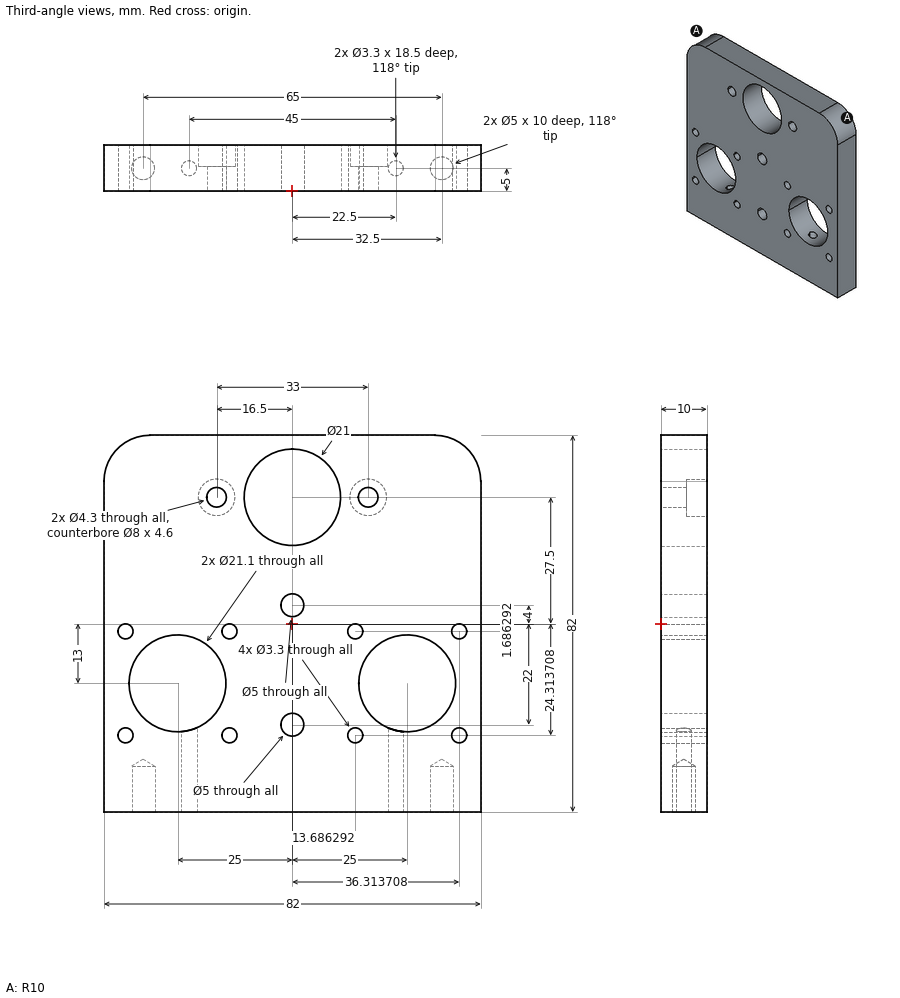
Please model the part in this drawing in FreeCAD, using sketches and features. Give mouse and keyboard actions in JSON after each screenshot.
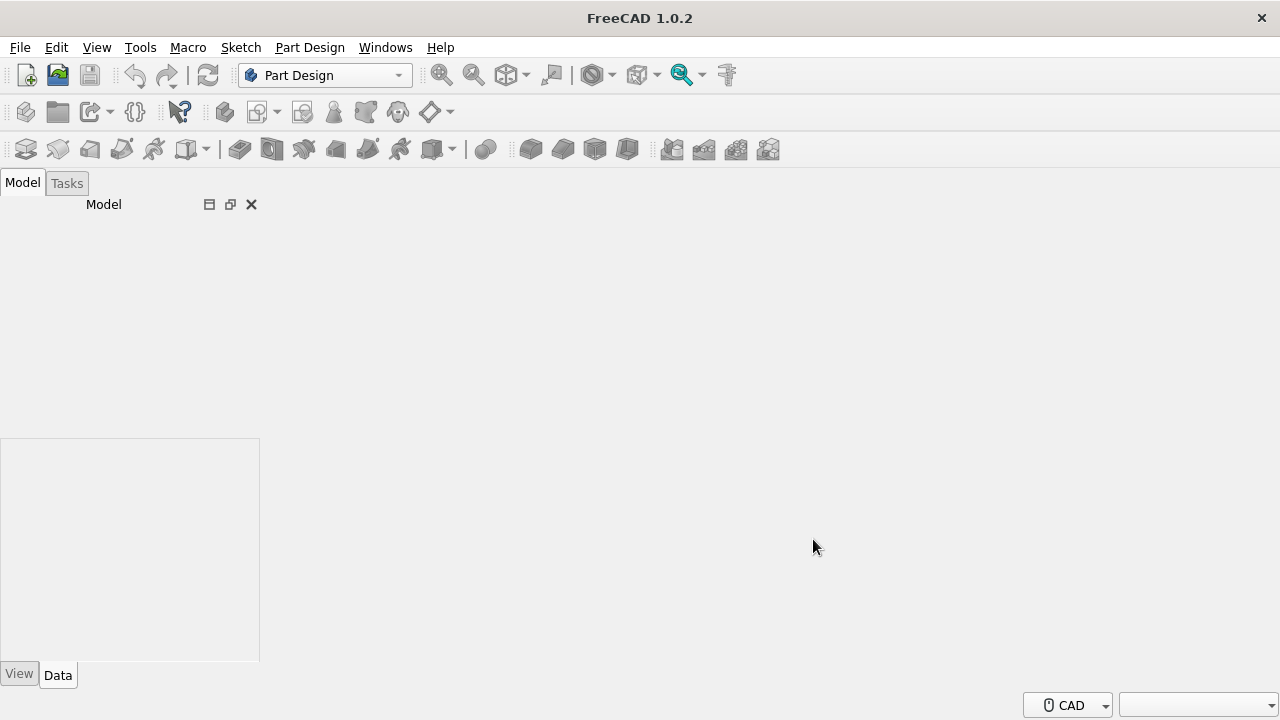
{"action": "left_click", "coordinate": [26, 76]}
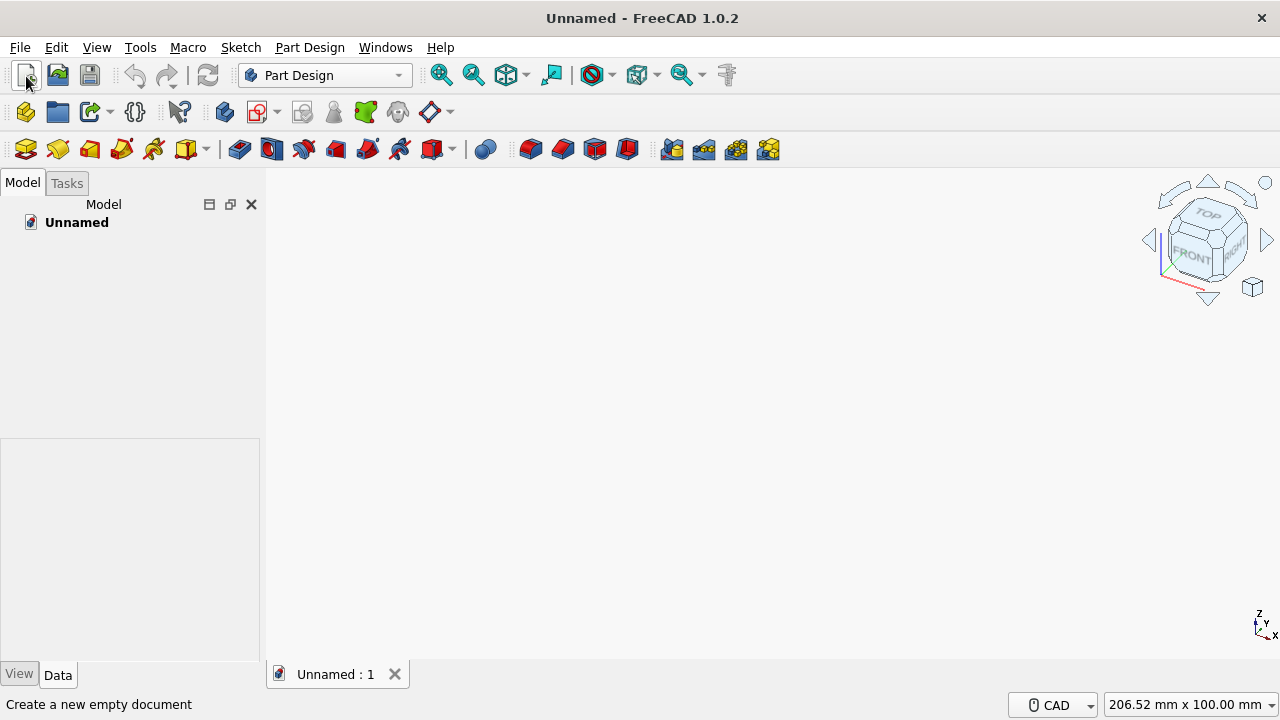
{"action": "left_click", "coordinate": [258, 112]}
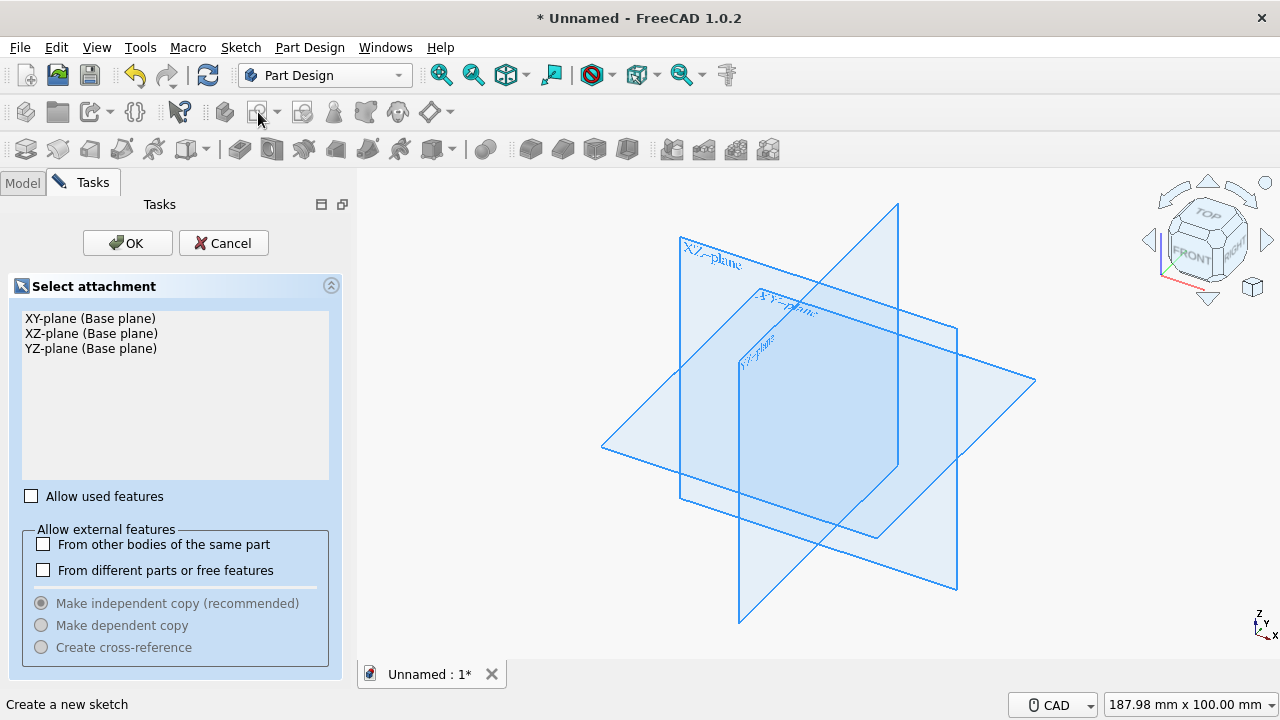
{"action": "left_click", "coordinate": [82, 334]}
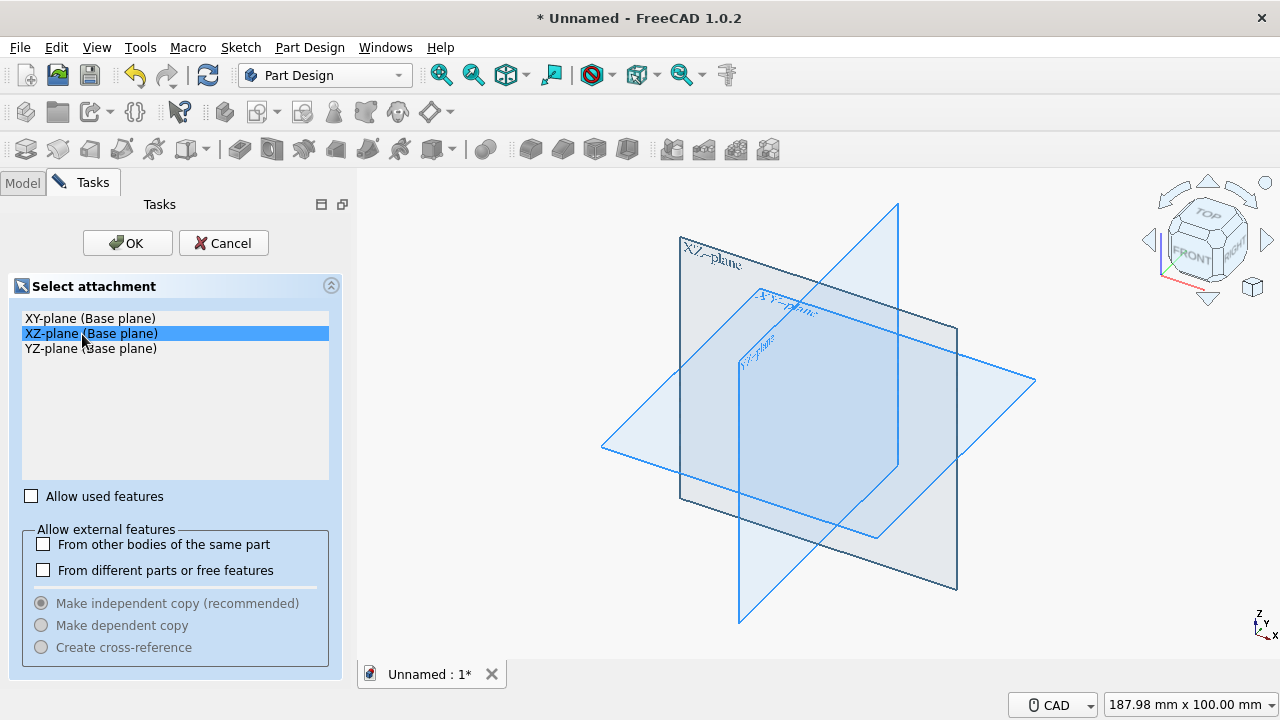
{"action": "left_click", "coordinate": [128, 243]}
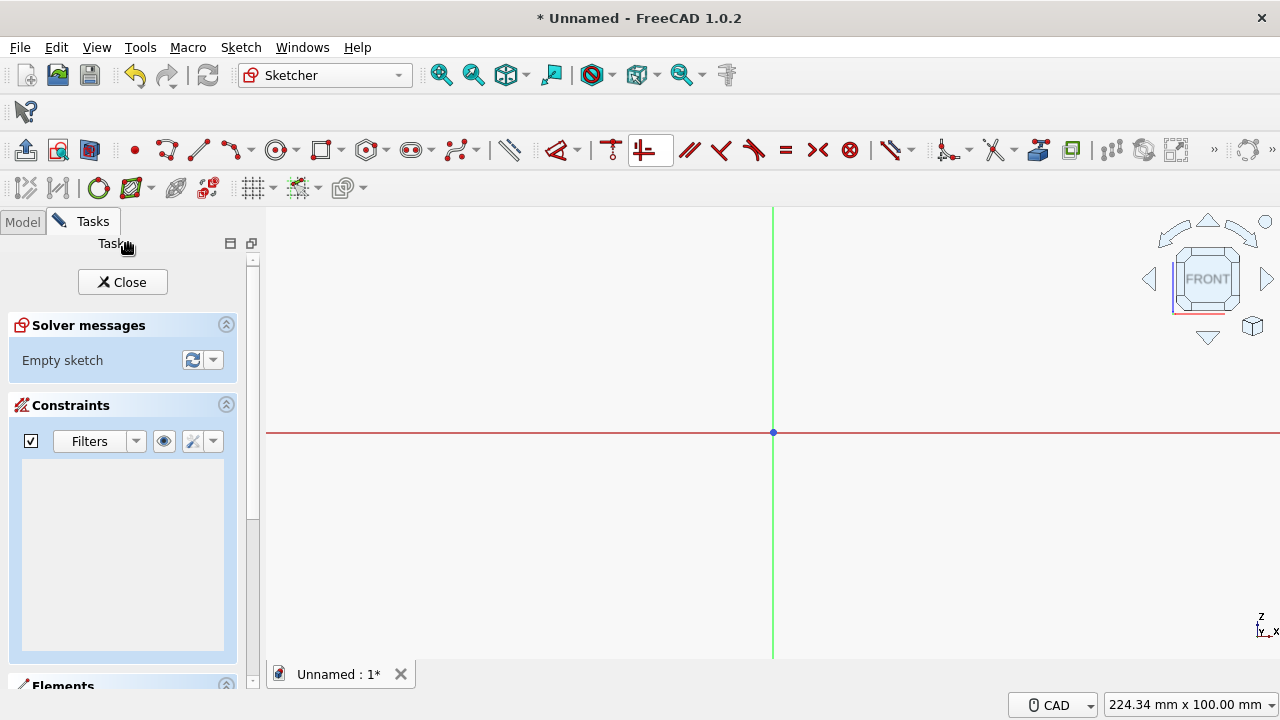
{"action": "scroll", "coordinate": [395, 433], "scroll_direction": "down", "scroll_amount": 1}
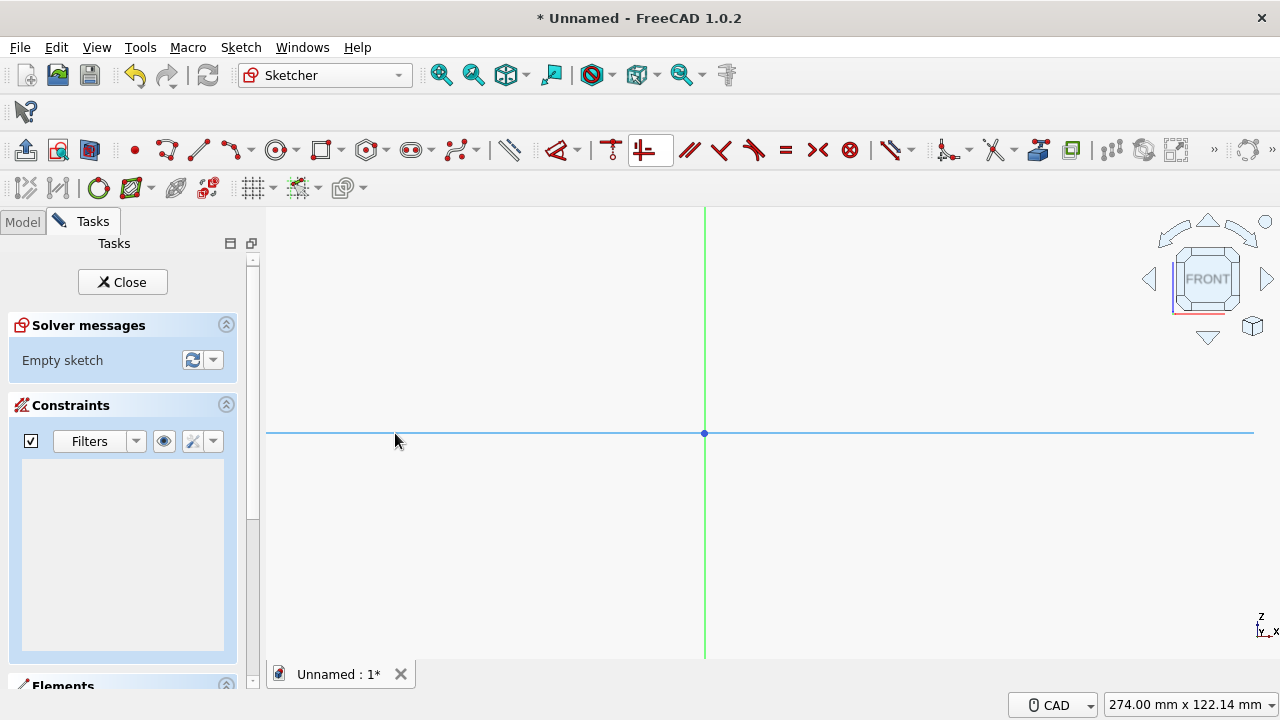
{"action": "key", "text": "g v"}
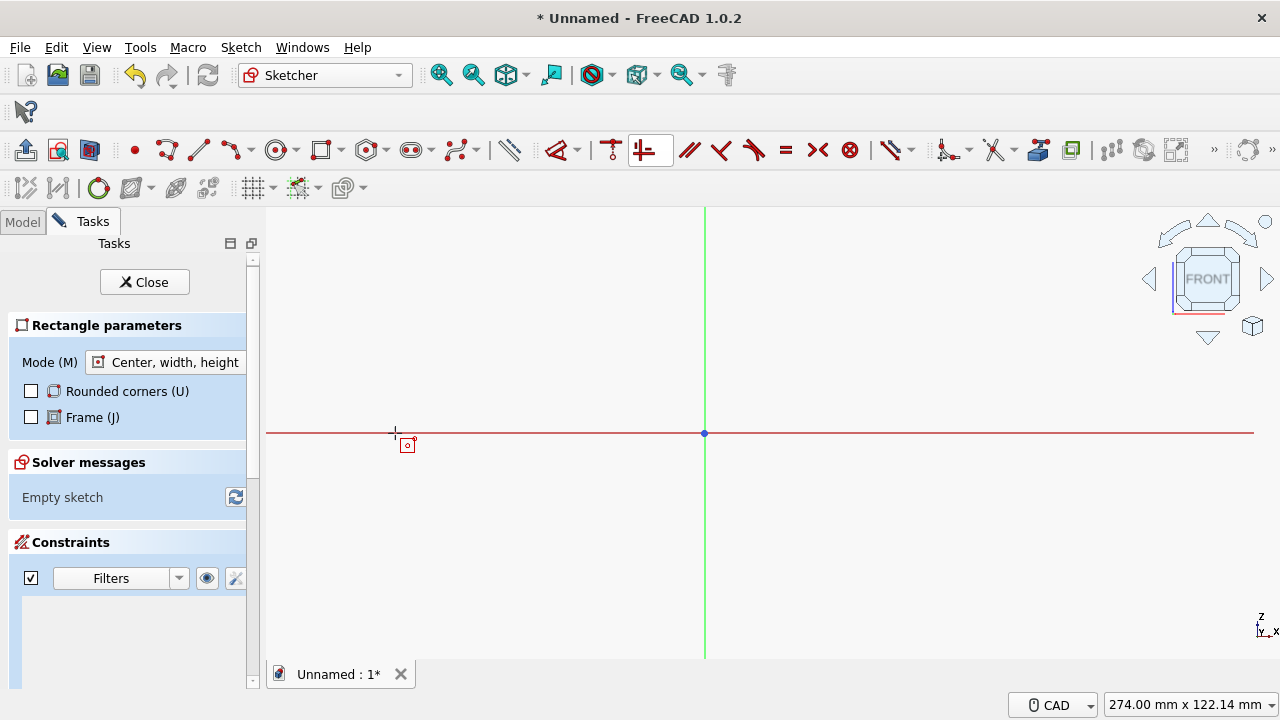
{"action": "left_click", "coordinate": [705, 433]}
{"action": "left_click", "coordinate": [856, 281]}
{"action": "key", "text": "Escape"}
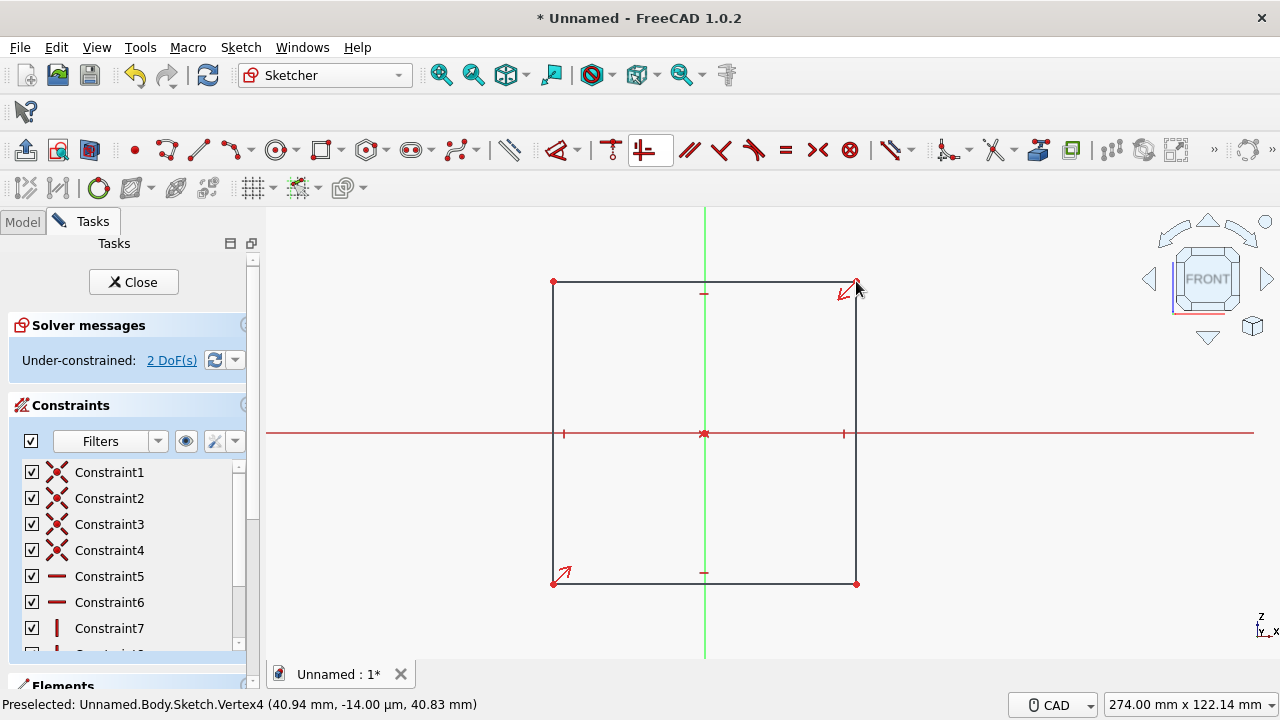
{"action": "left_click", "coordinate": [644, 584]}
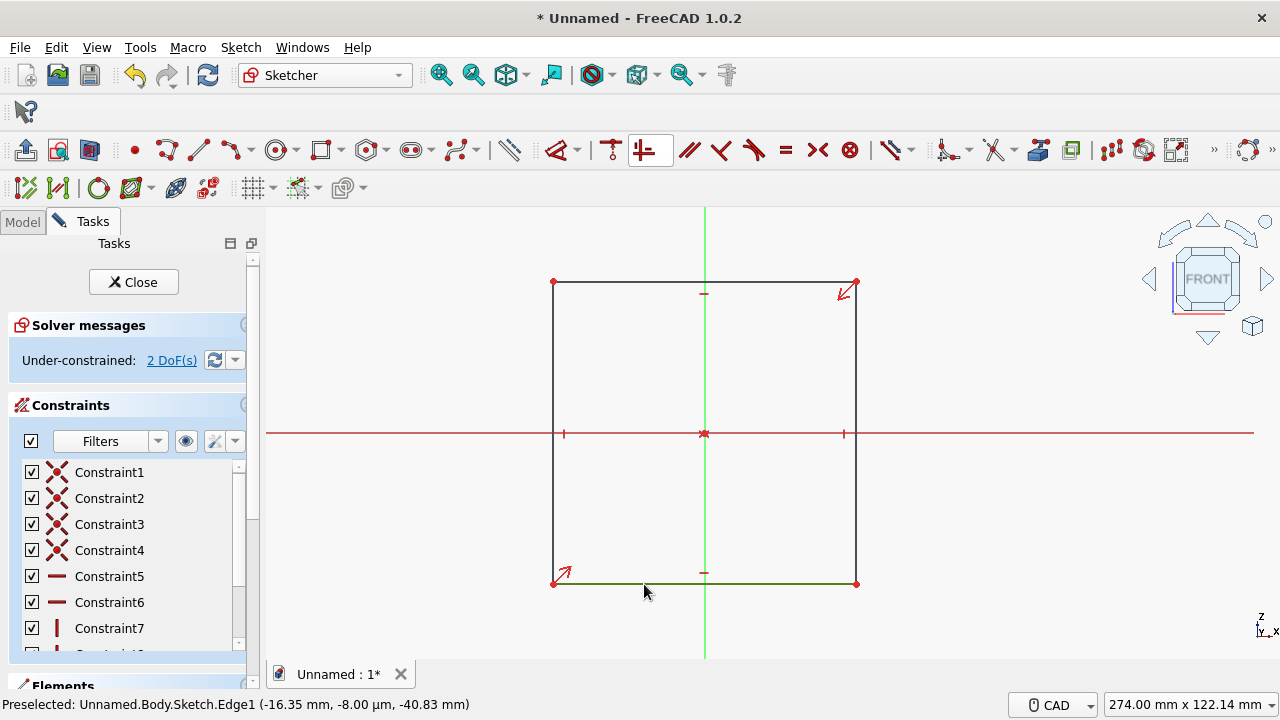
{"action": "left_click", "coordinate": [580, 150]}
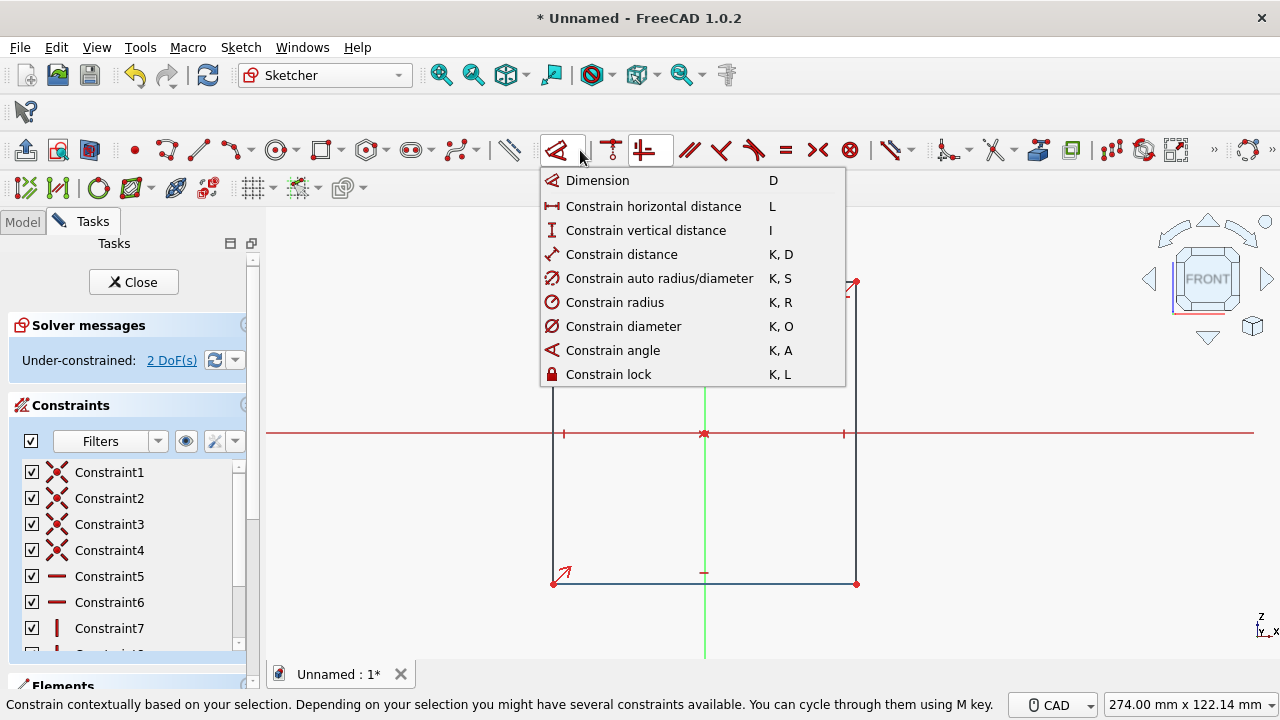
{"action": "left_click", "coordinate": [693, 206]}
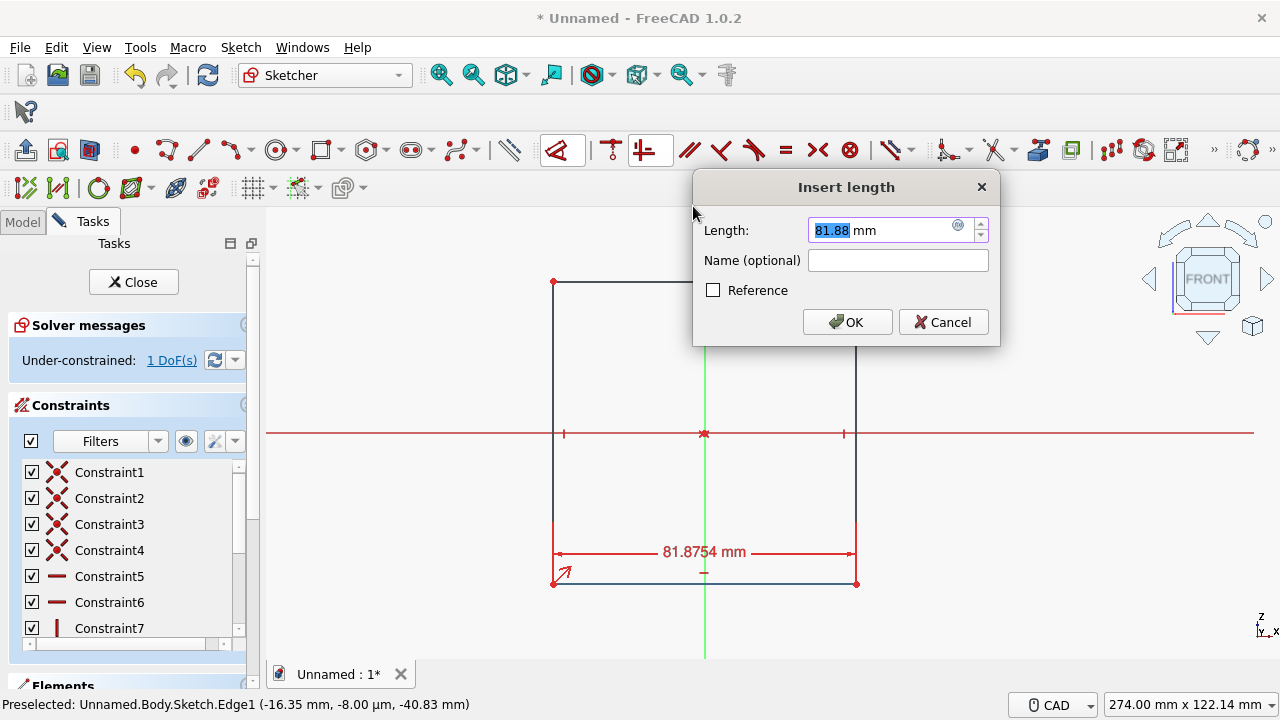
{"action": "type", "text": "82"}
{"action": "key", "text": "Return"}